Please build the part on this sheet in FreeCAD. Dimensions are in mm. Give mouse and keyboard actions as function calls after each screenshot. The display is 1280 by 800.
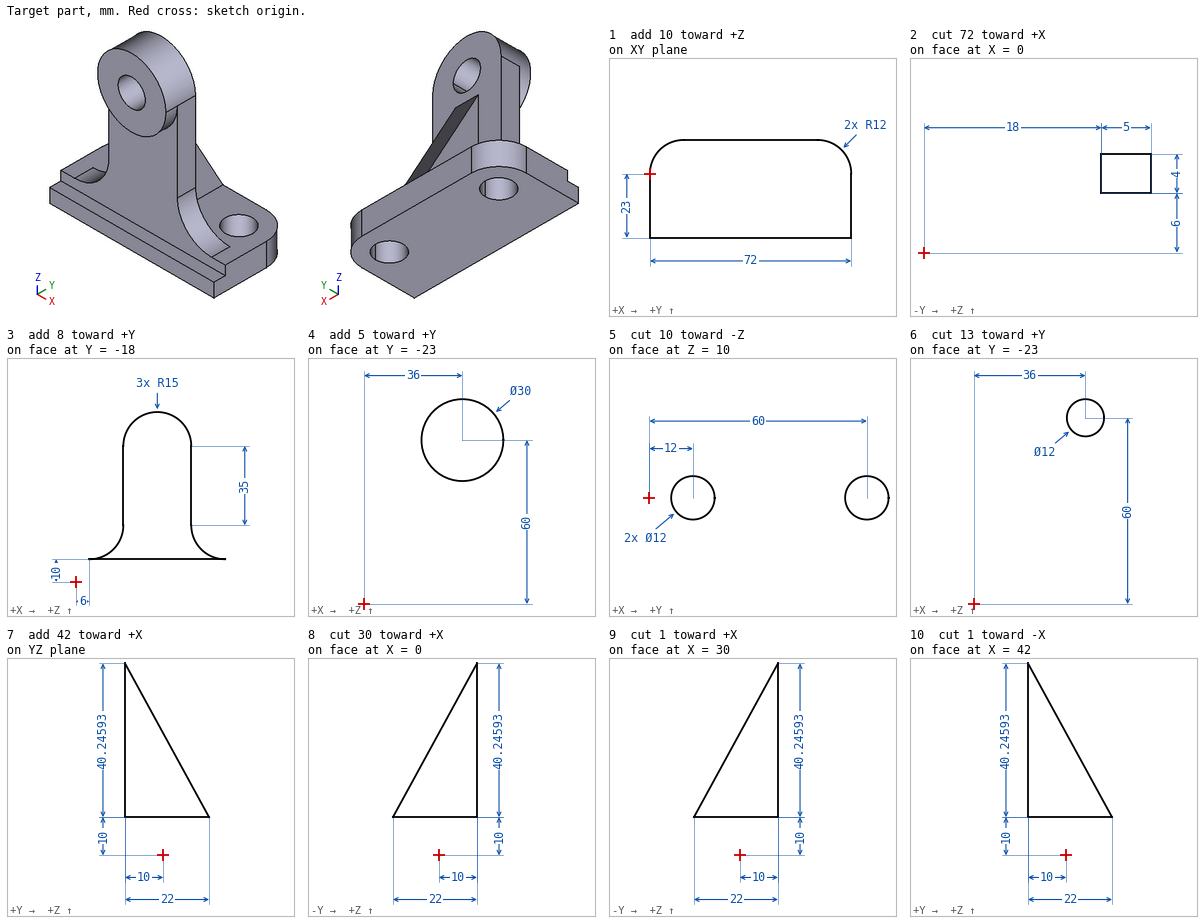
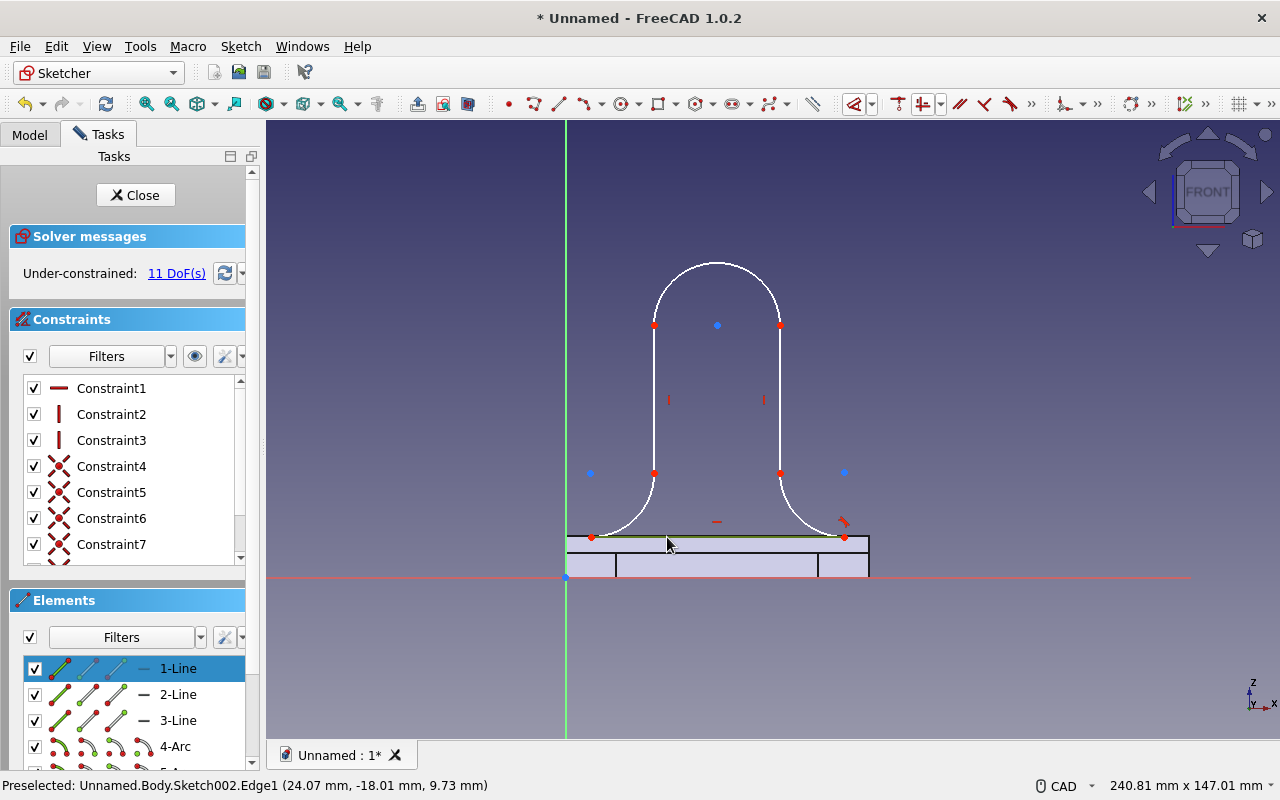
click(647, 503)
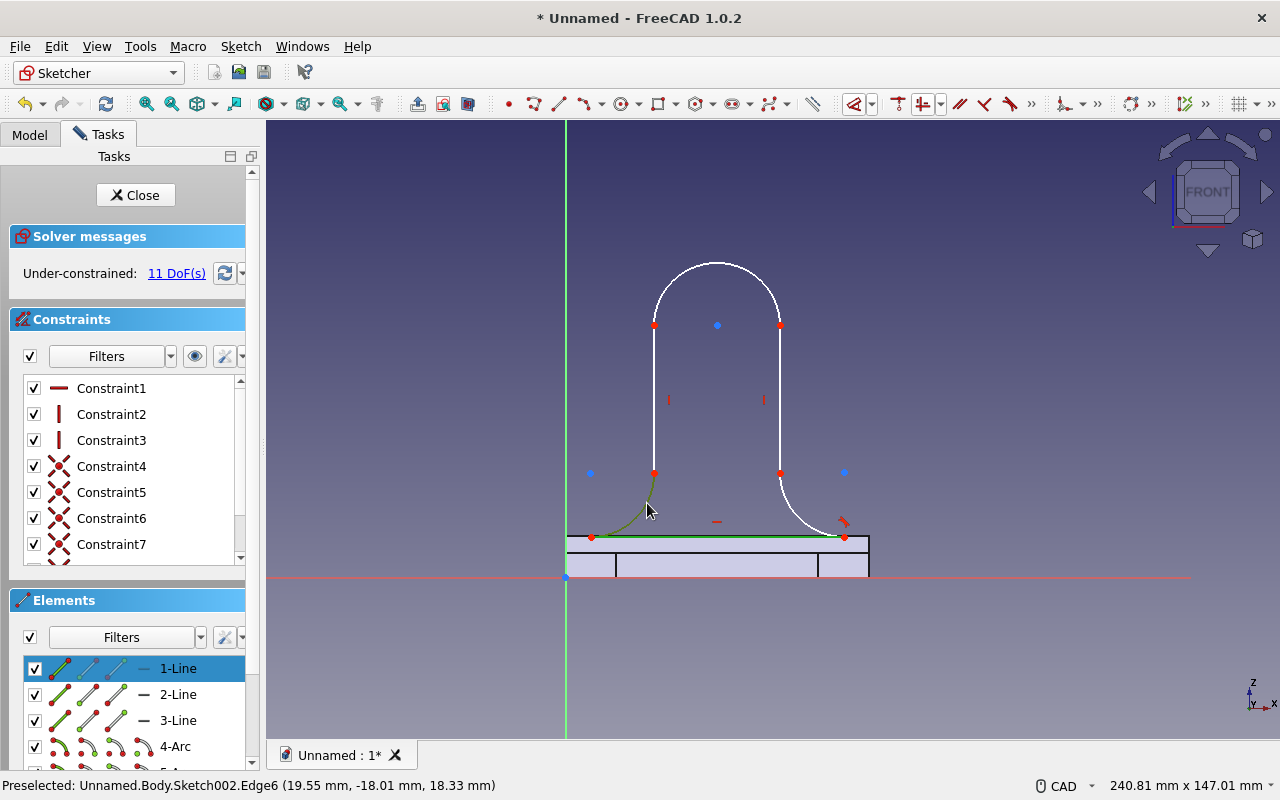
click(1010, 104)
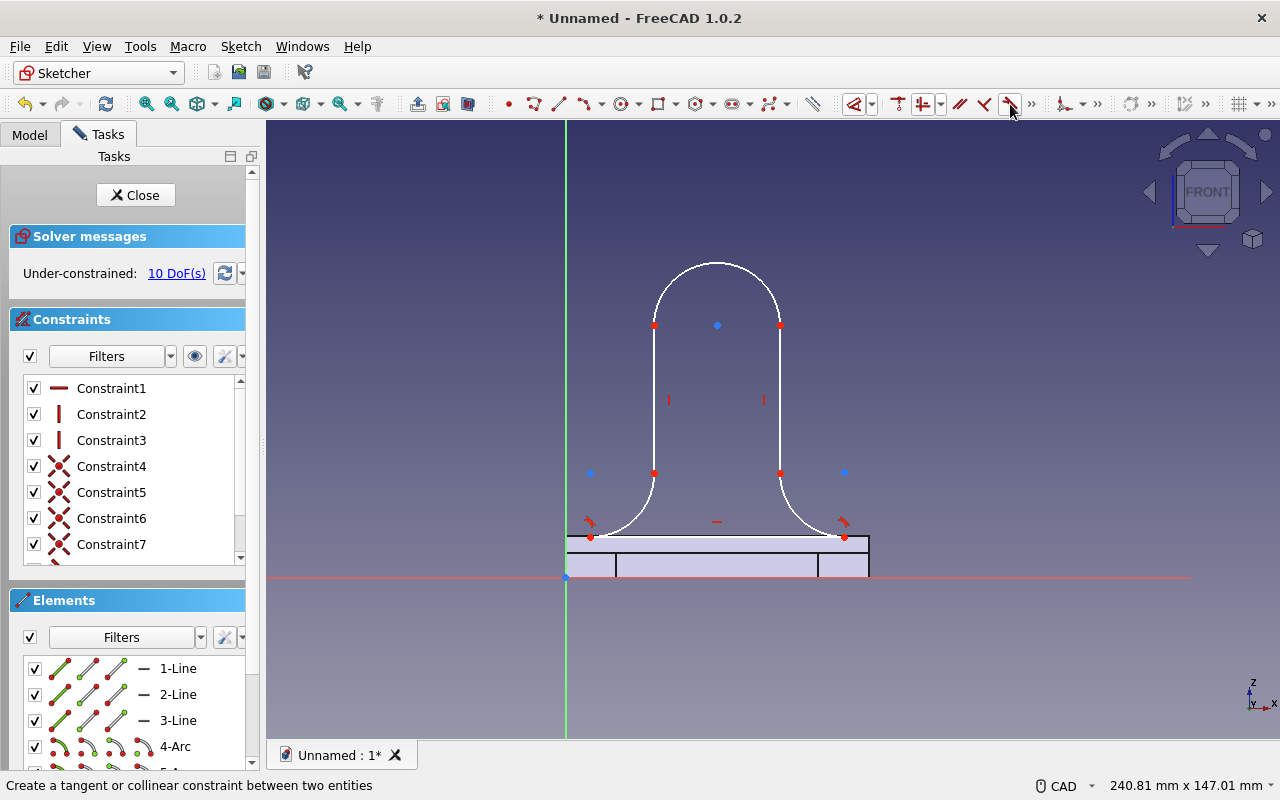
click(780, 430)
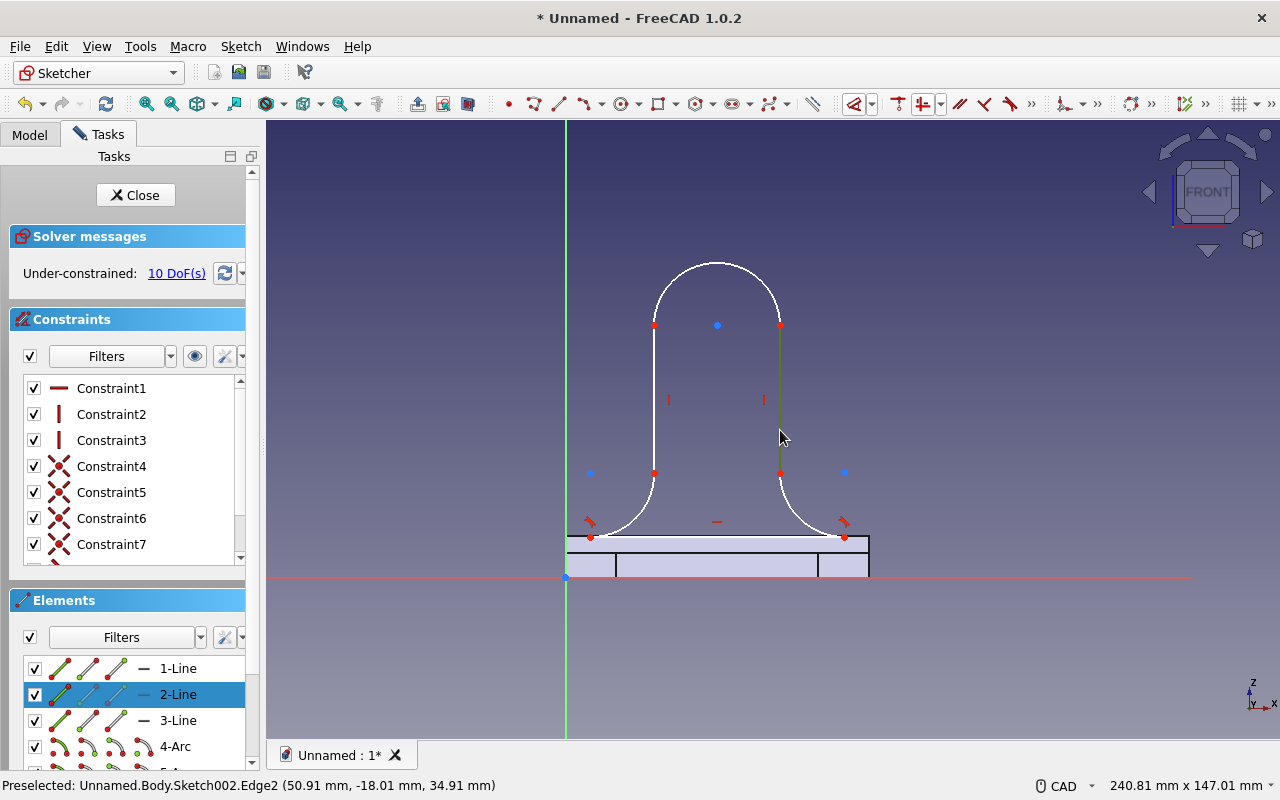
click(788, 503)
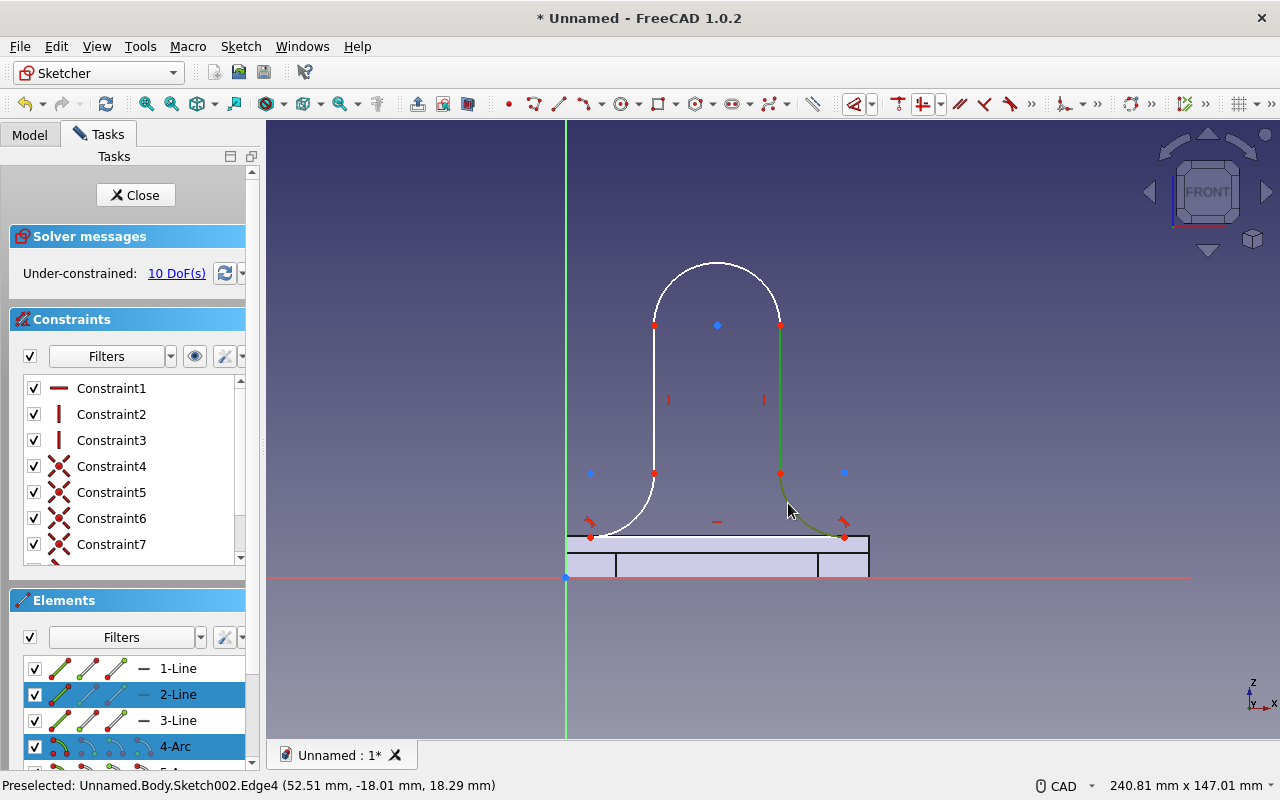
click(1010, 104)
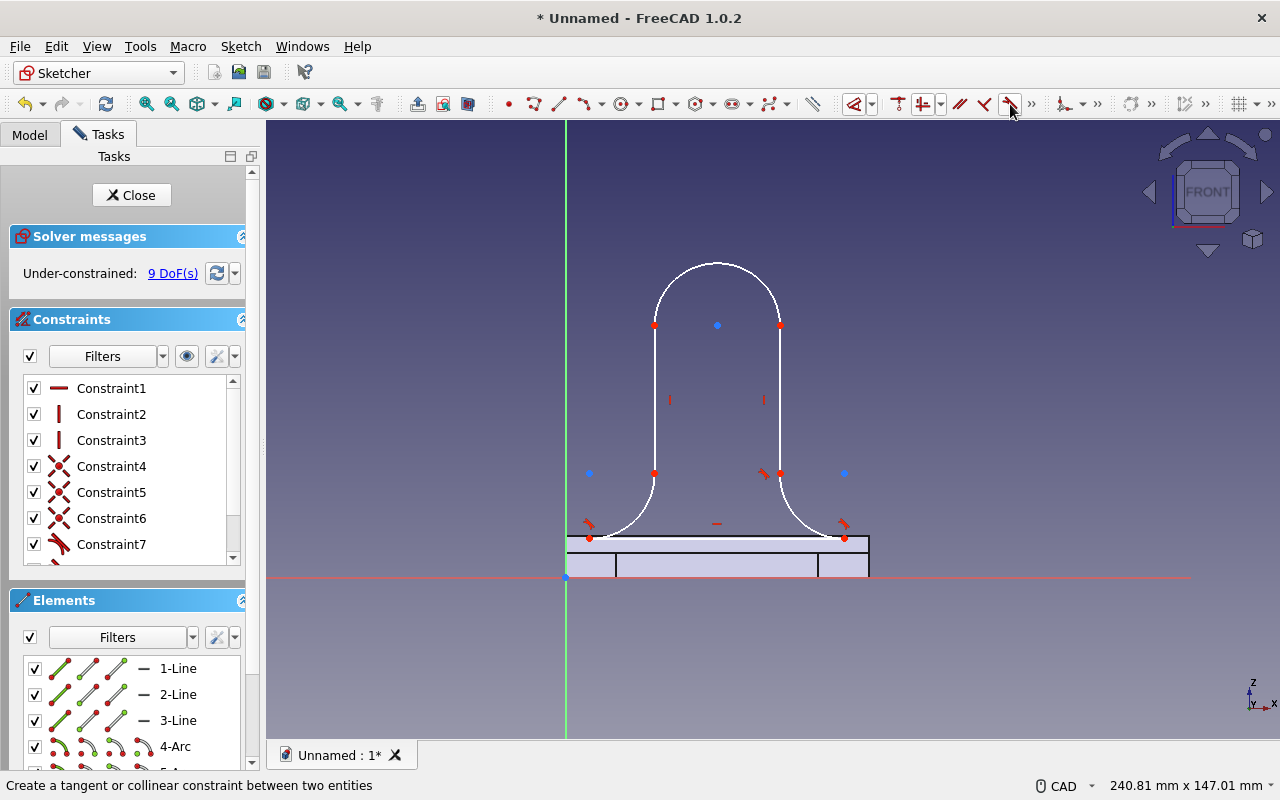
click(780, 430)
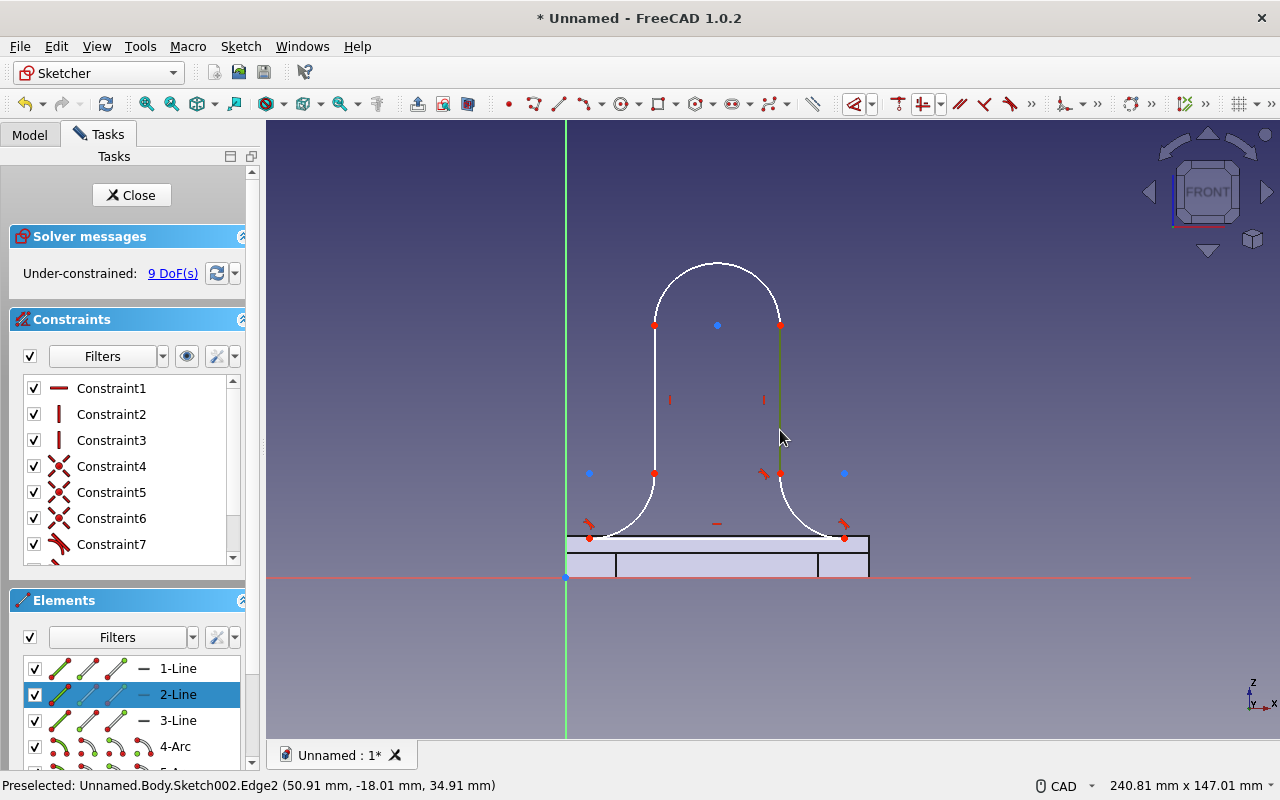
click(754, 275)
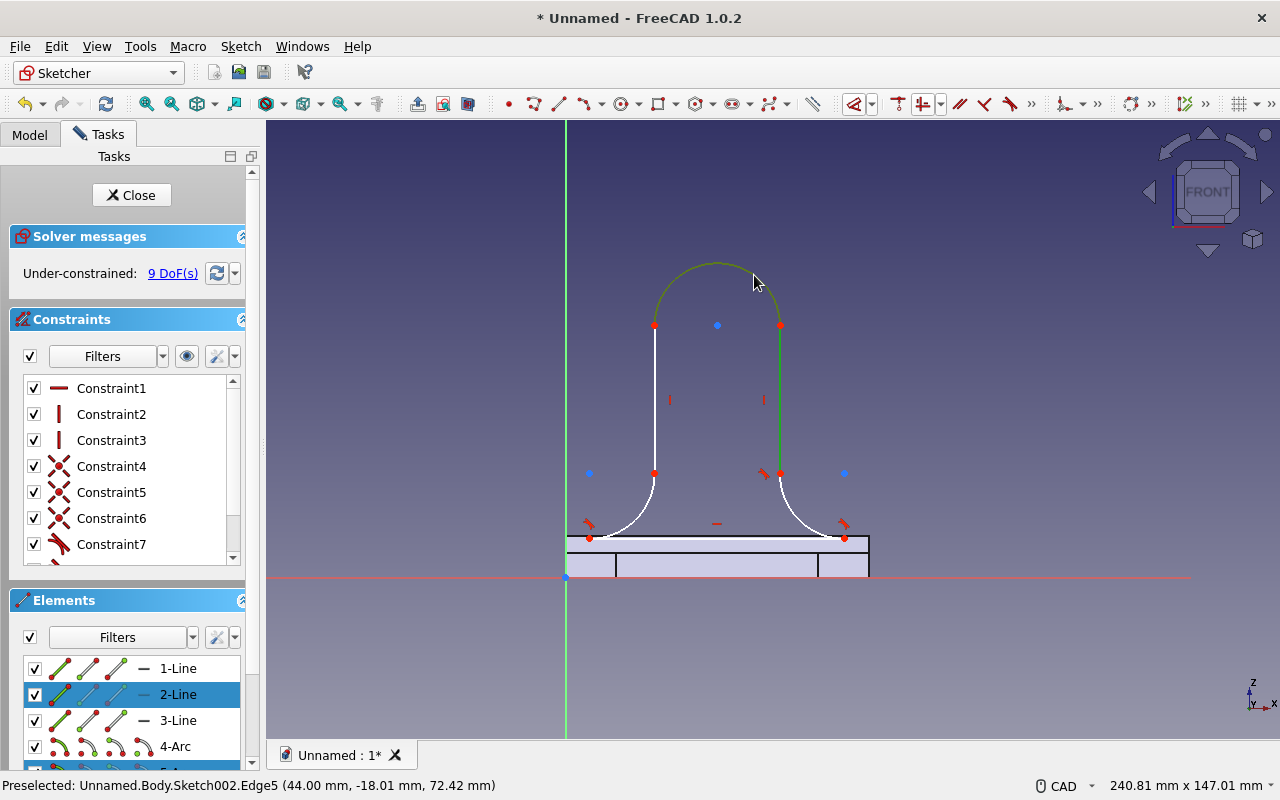
click(1010, 104)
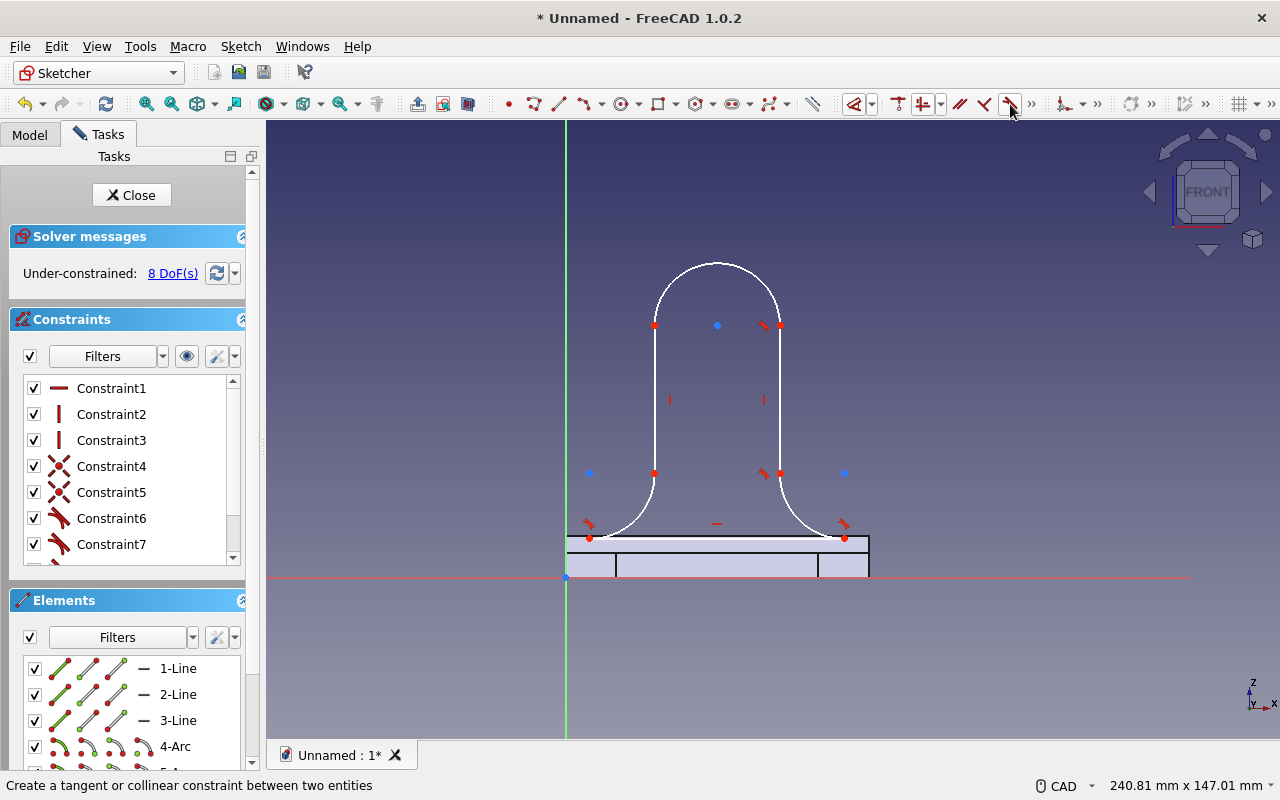
click(655, 370)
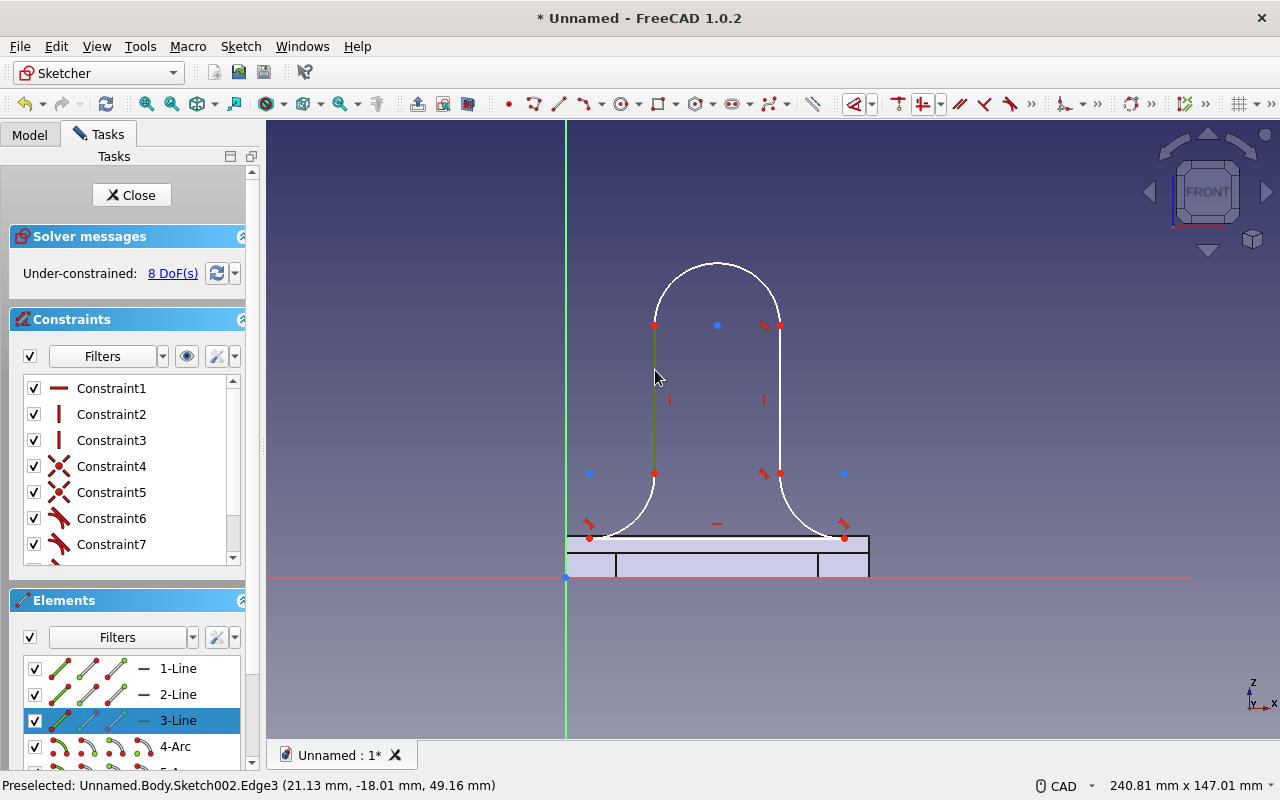
click(754, 275)